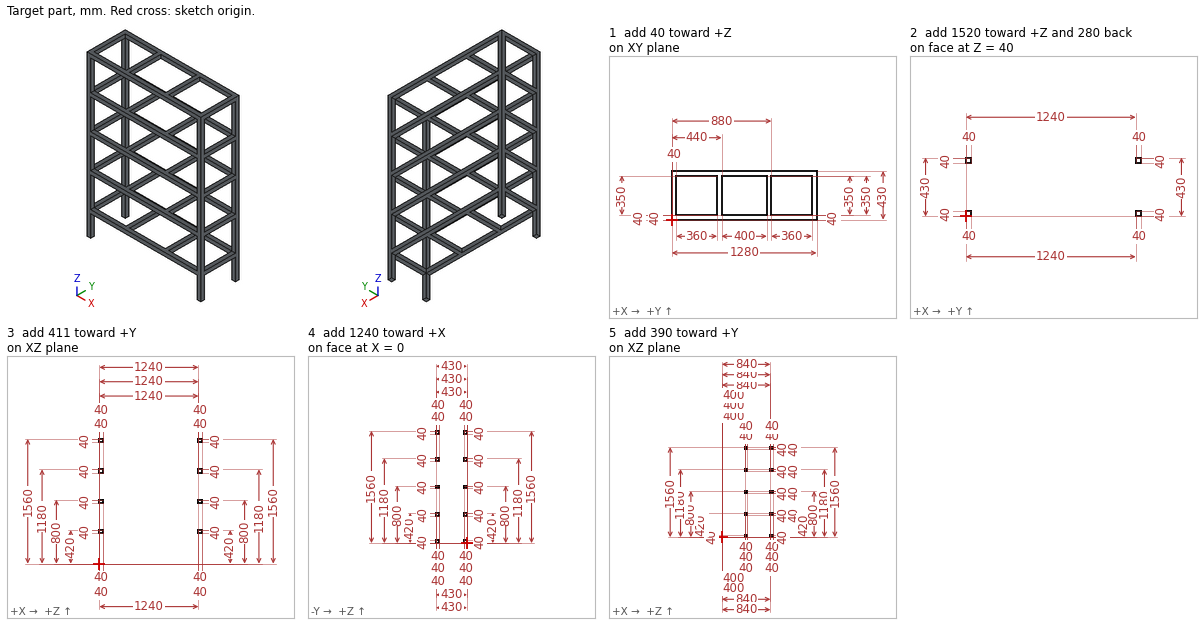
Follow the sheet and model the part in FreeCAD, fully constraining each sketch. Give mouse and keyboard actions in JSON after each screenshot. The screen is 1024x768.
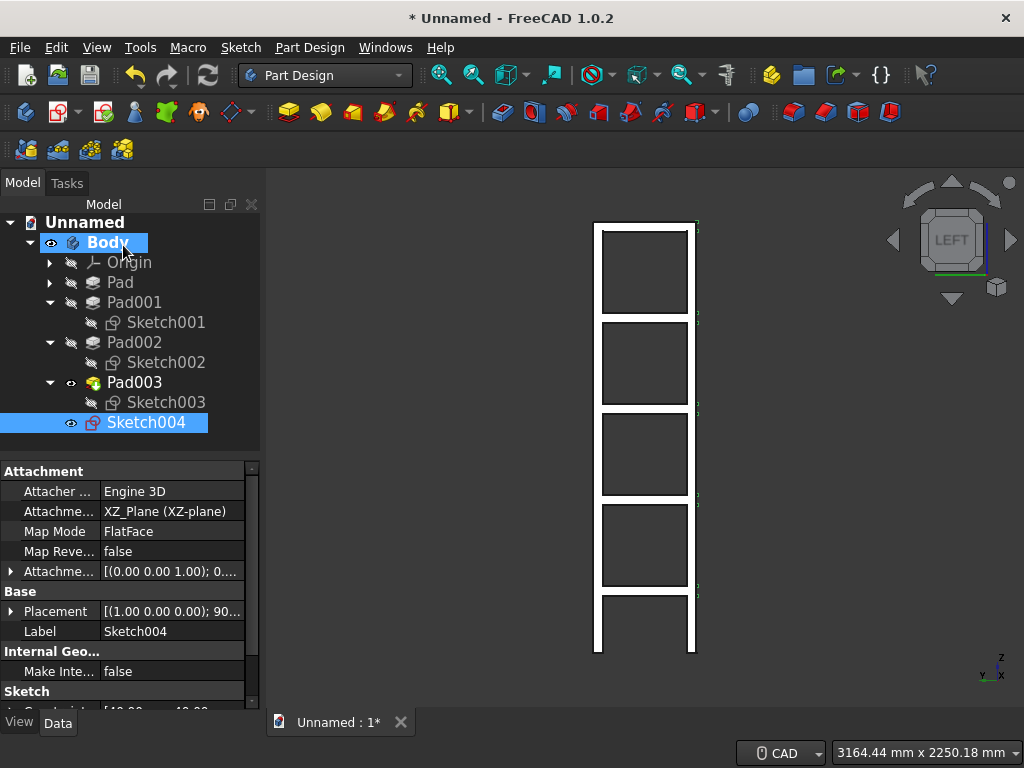
{"action": "left_click", "coordinate": [290, 112]}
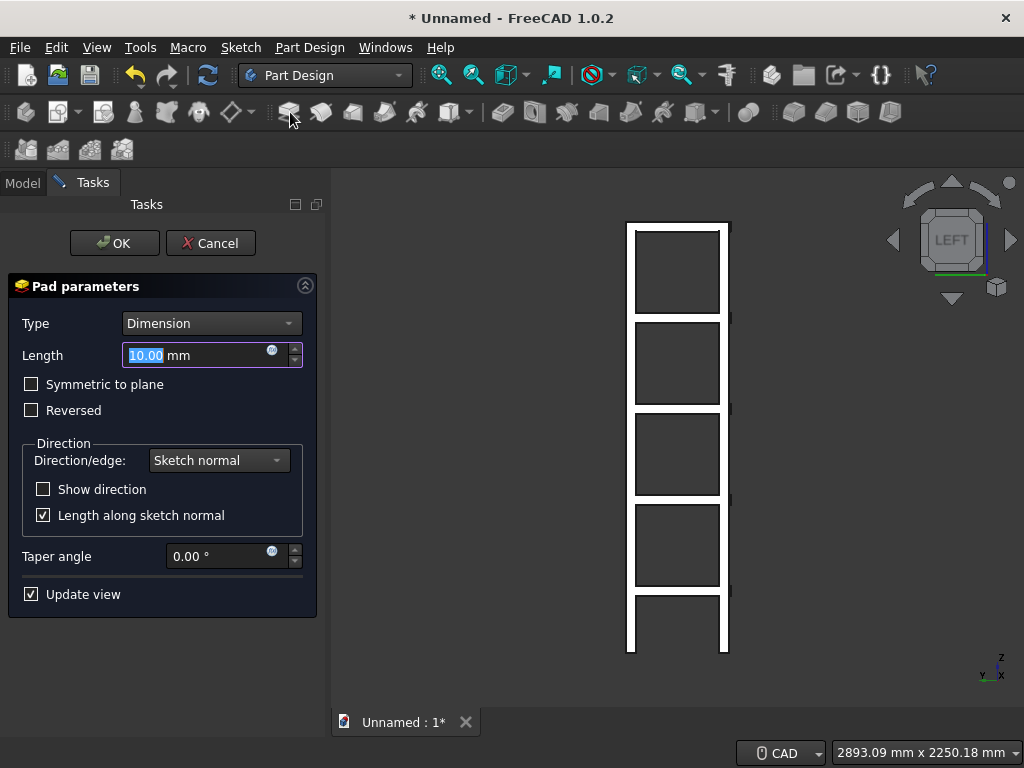
{"action": "type", "text": "390"}
{"action": "key", "text": "Tab"}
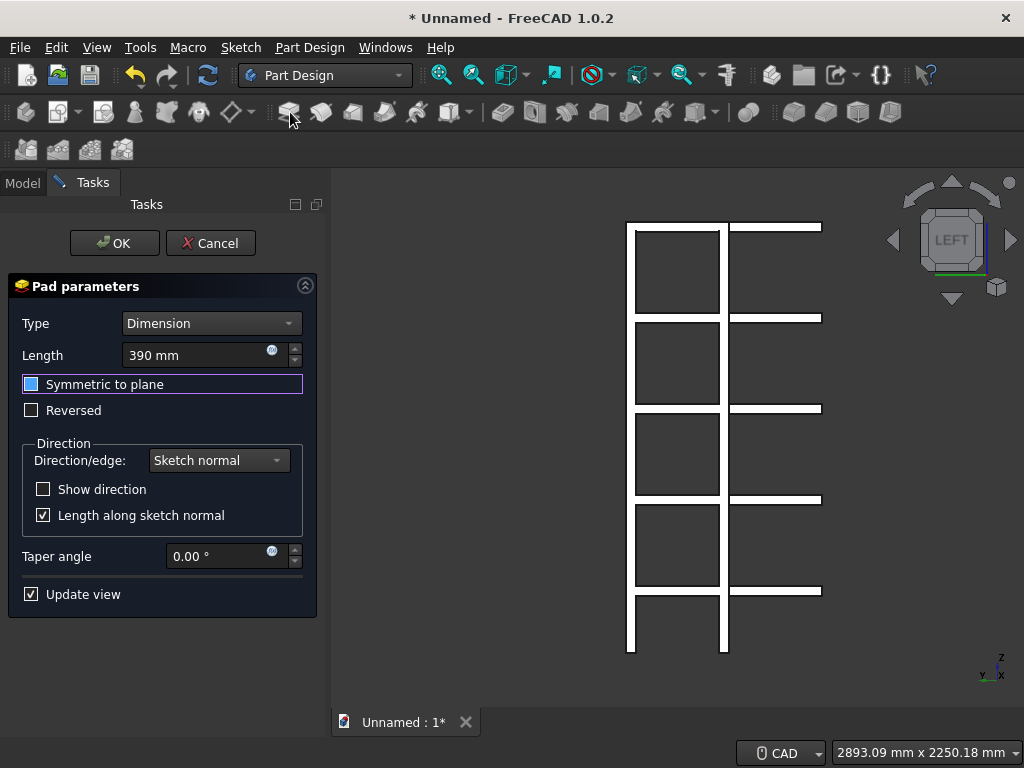
{"action": "left_click", "coordinate": [30, 410]}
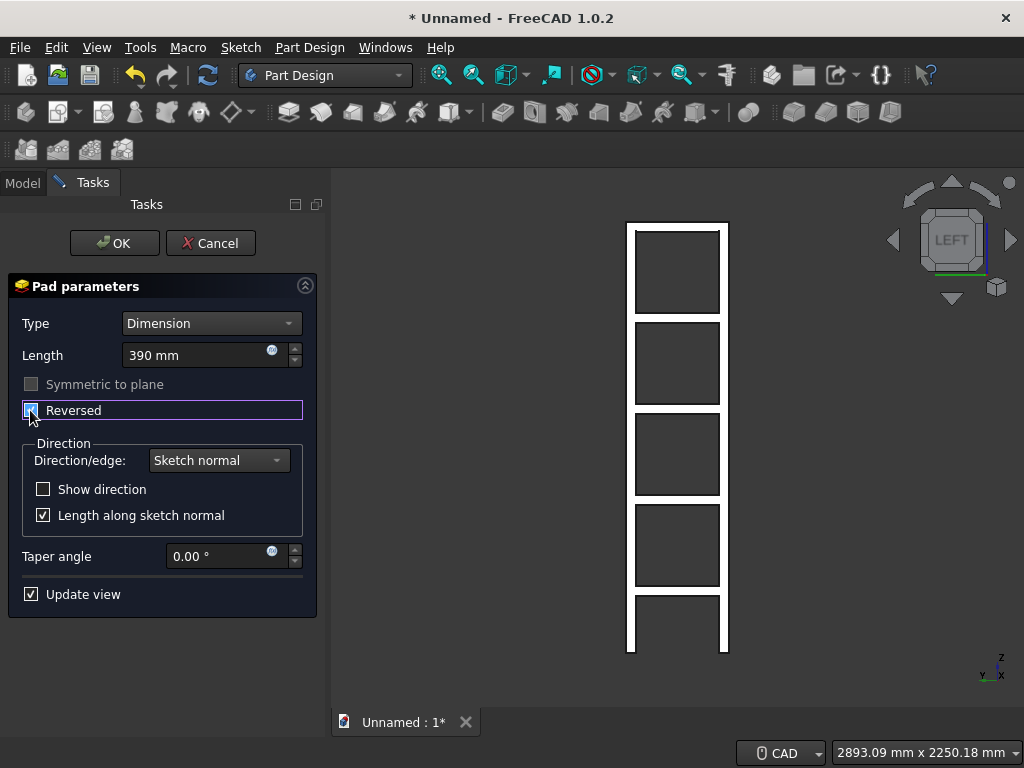
{"action": "left_click", "coordinate": [115, 243]}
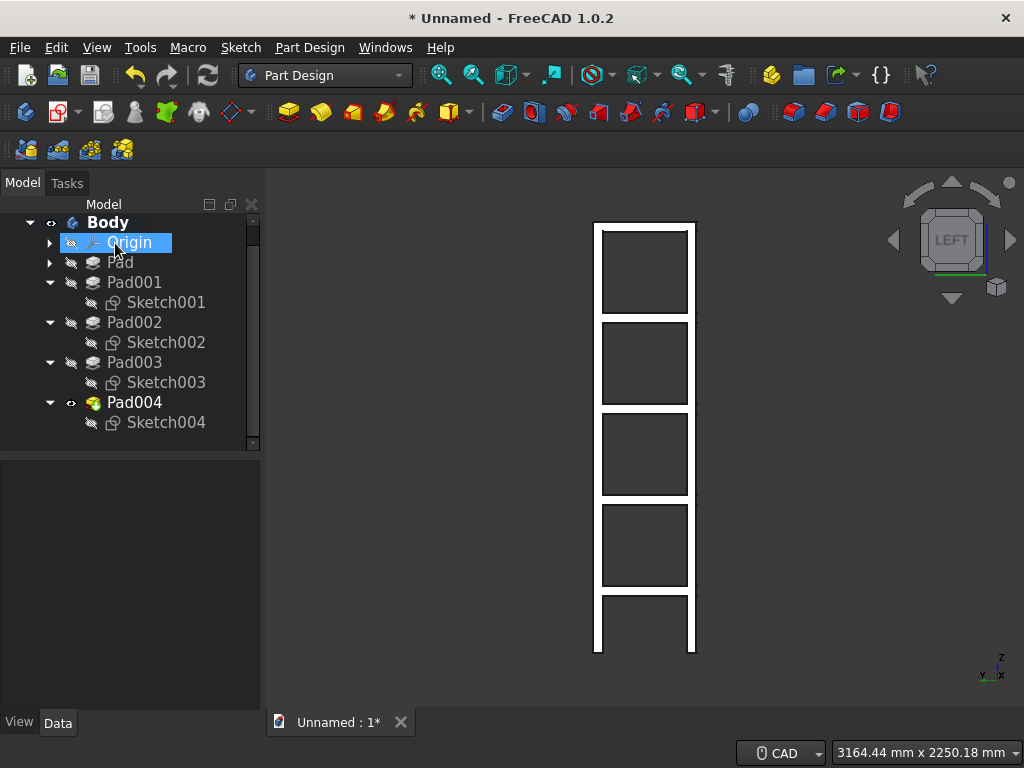
{"action": "key", "text": "0"}